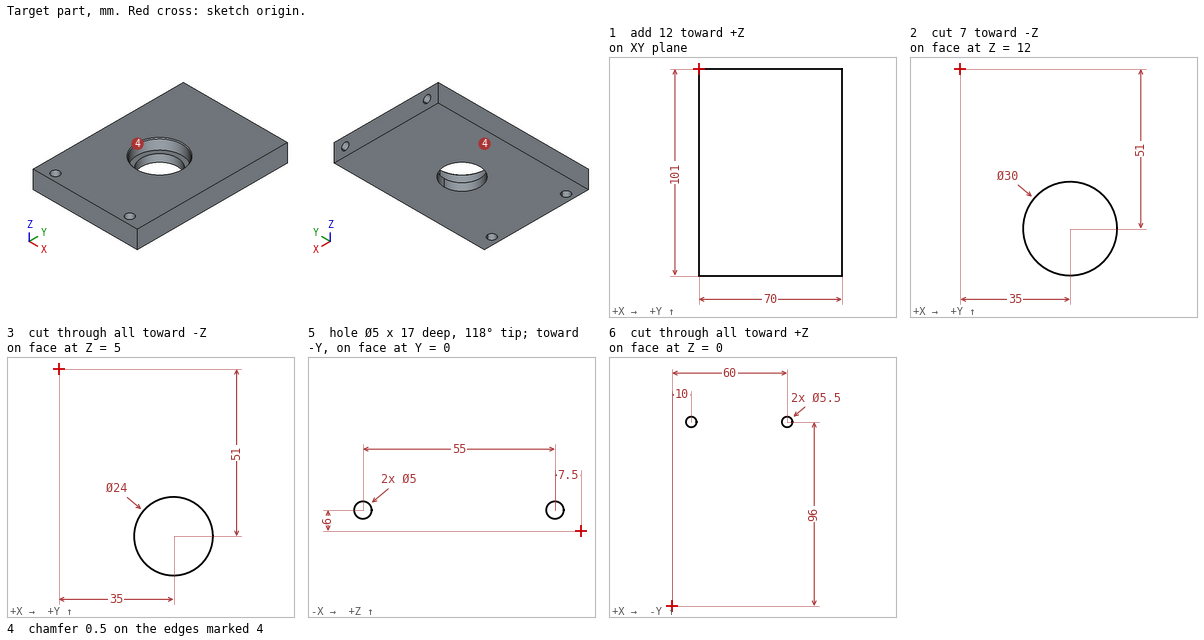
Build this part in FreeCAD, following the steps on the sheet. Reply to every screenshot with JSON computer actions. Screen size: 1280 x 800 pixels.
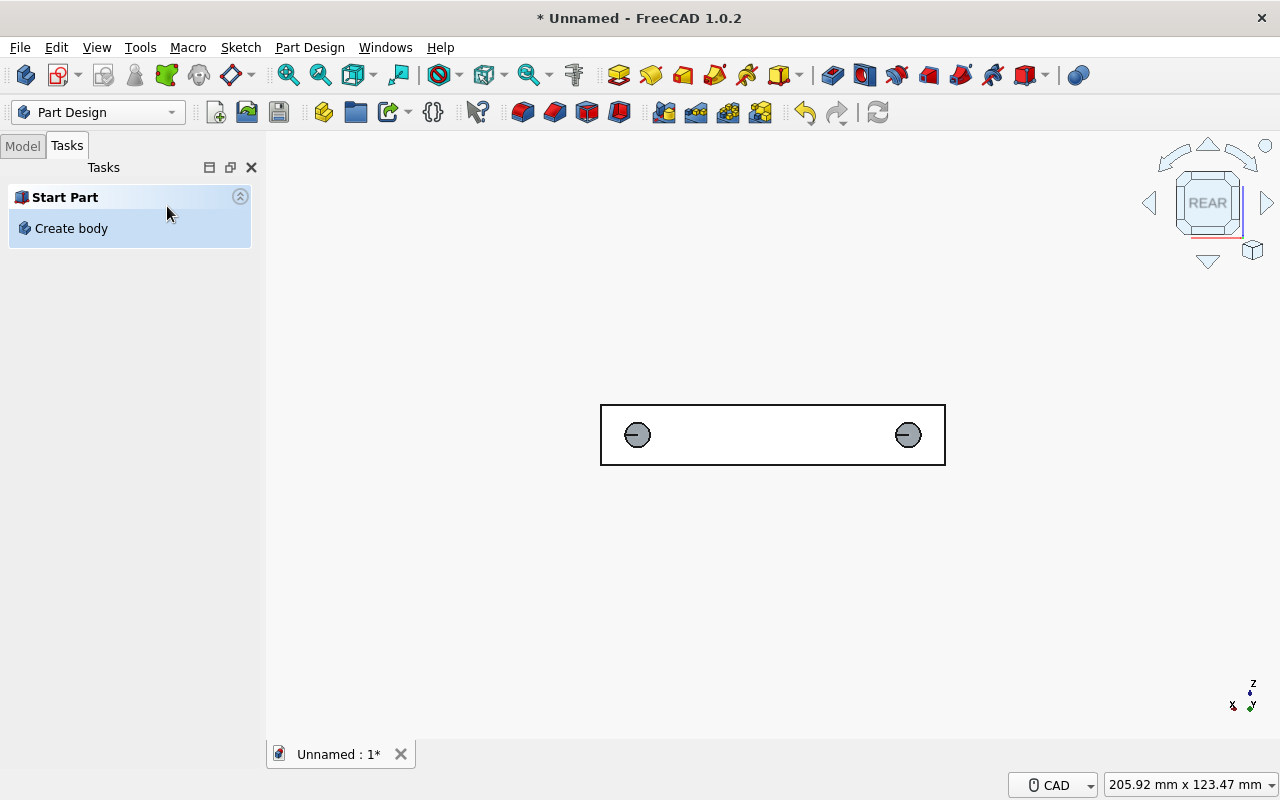
{"action": "left_click", "coordinate": [290, 76]}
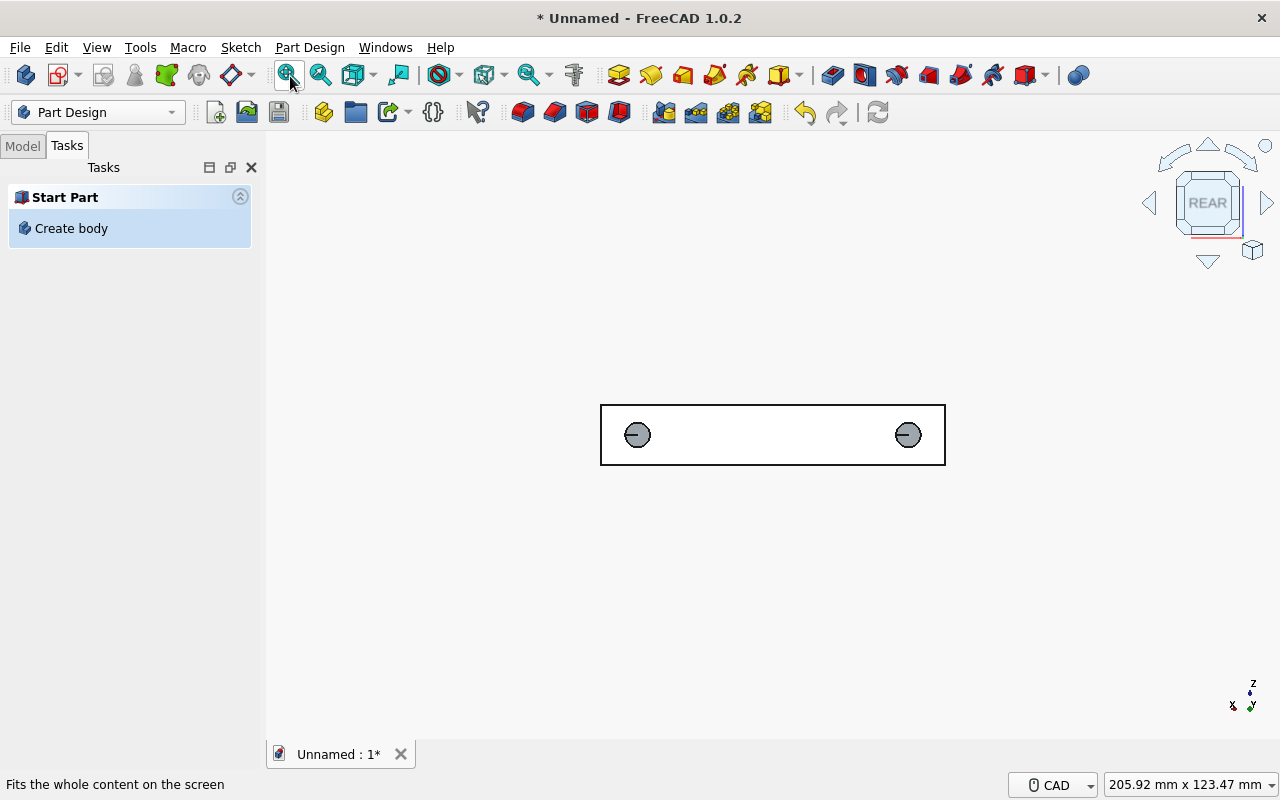
{"action": "key", "text": "5"}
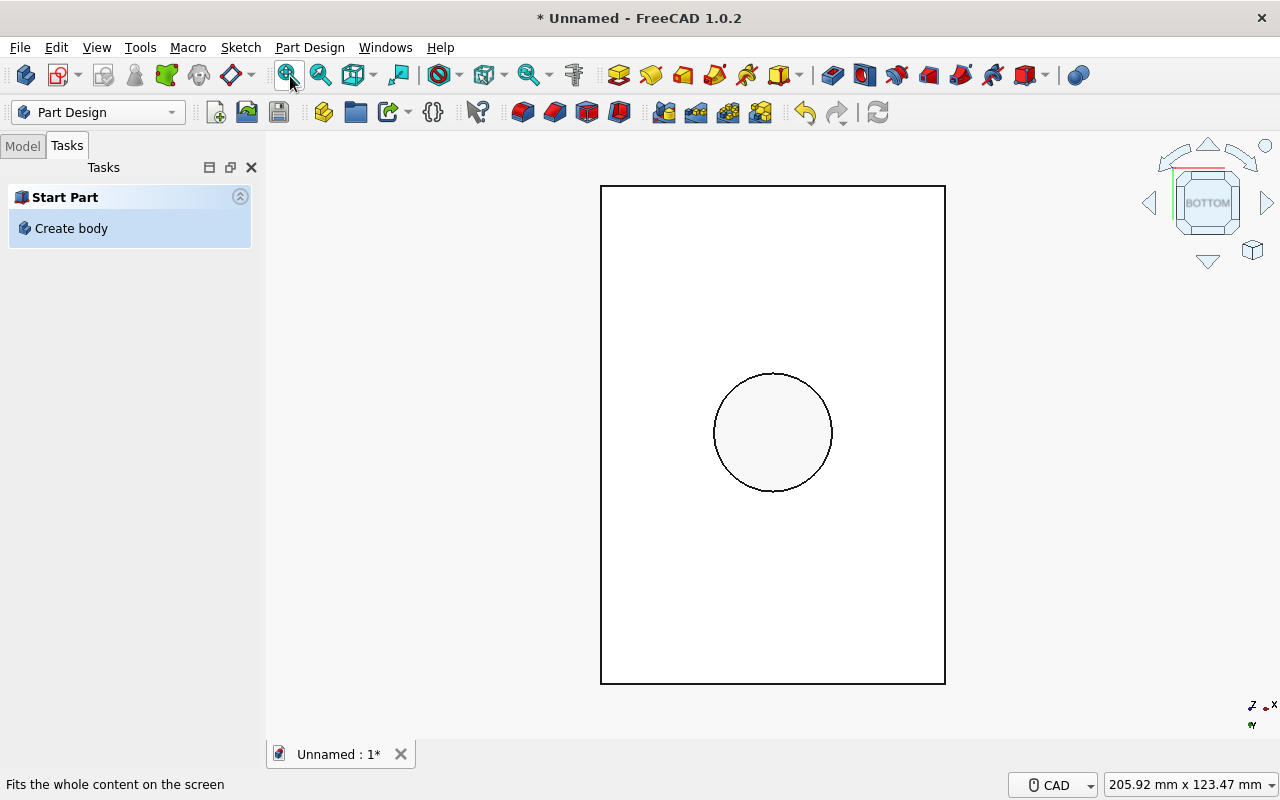
{"action": "left_click", "coordinate": [822, 576]}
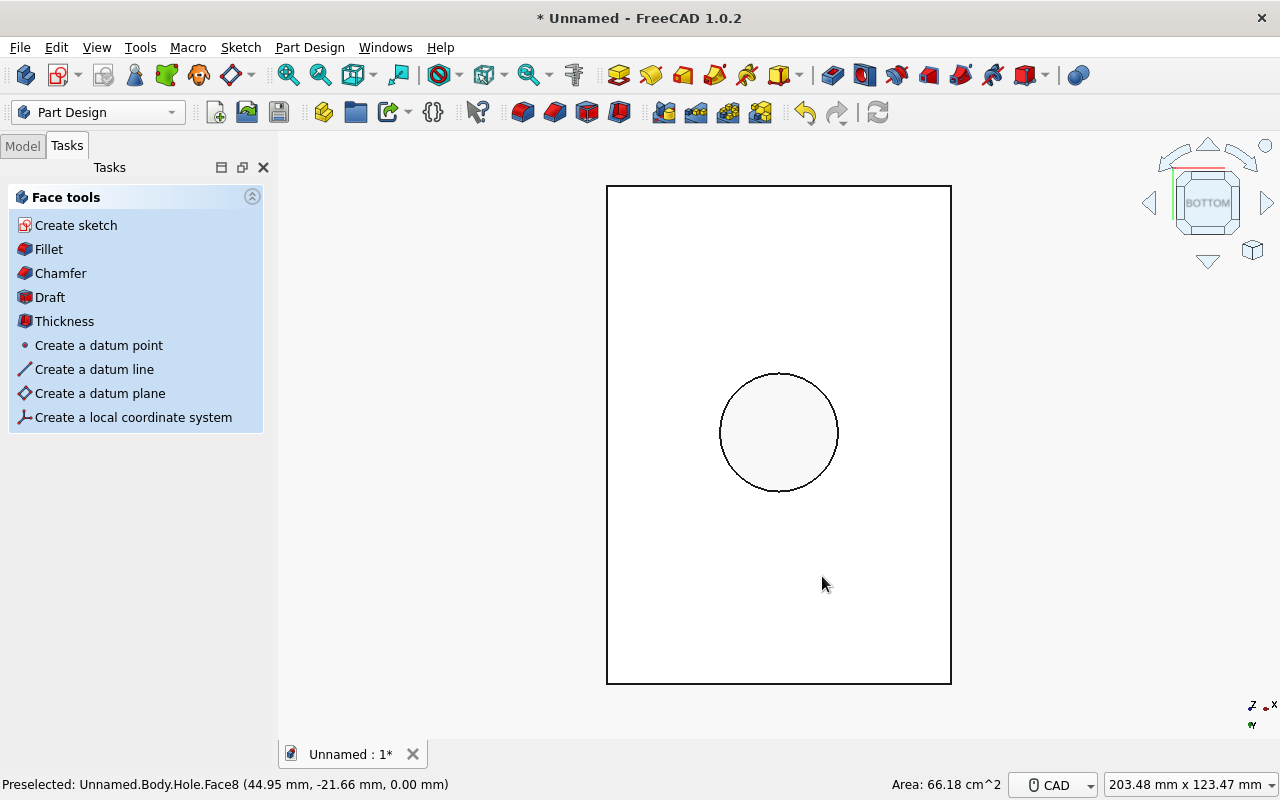
{"action": "left_click", "coordinate": [58, 76]}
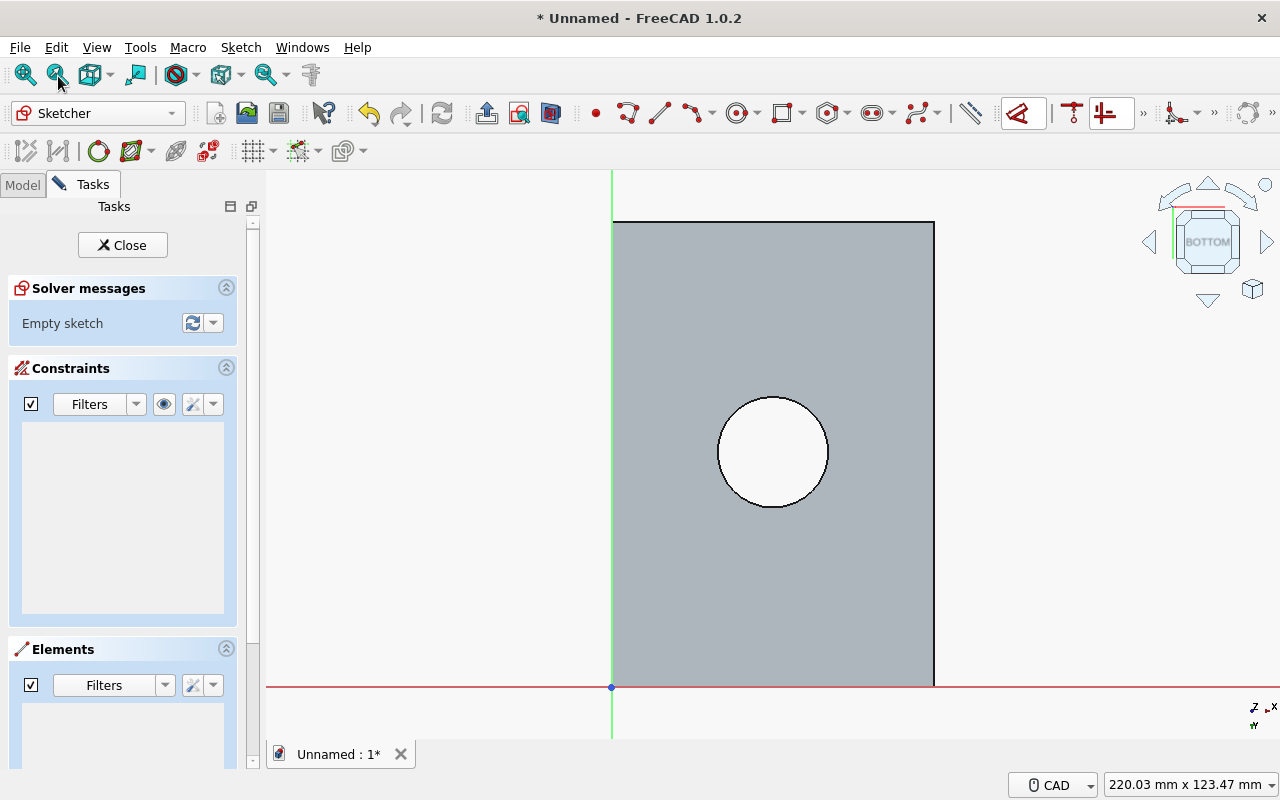
{"action": "scroll", "coordinate": [471, 431], "scroll_direction": "down", "scroll_amount": 1}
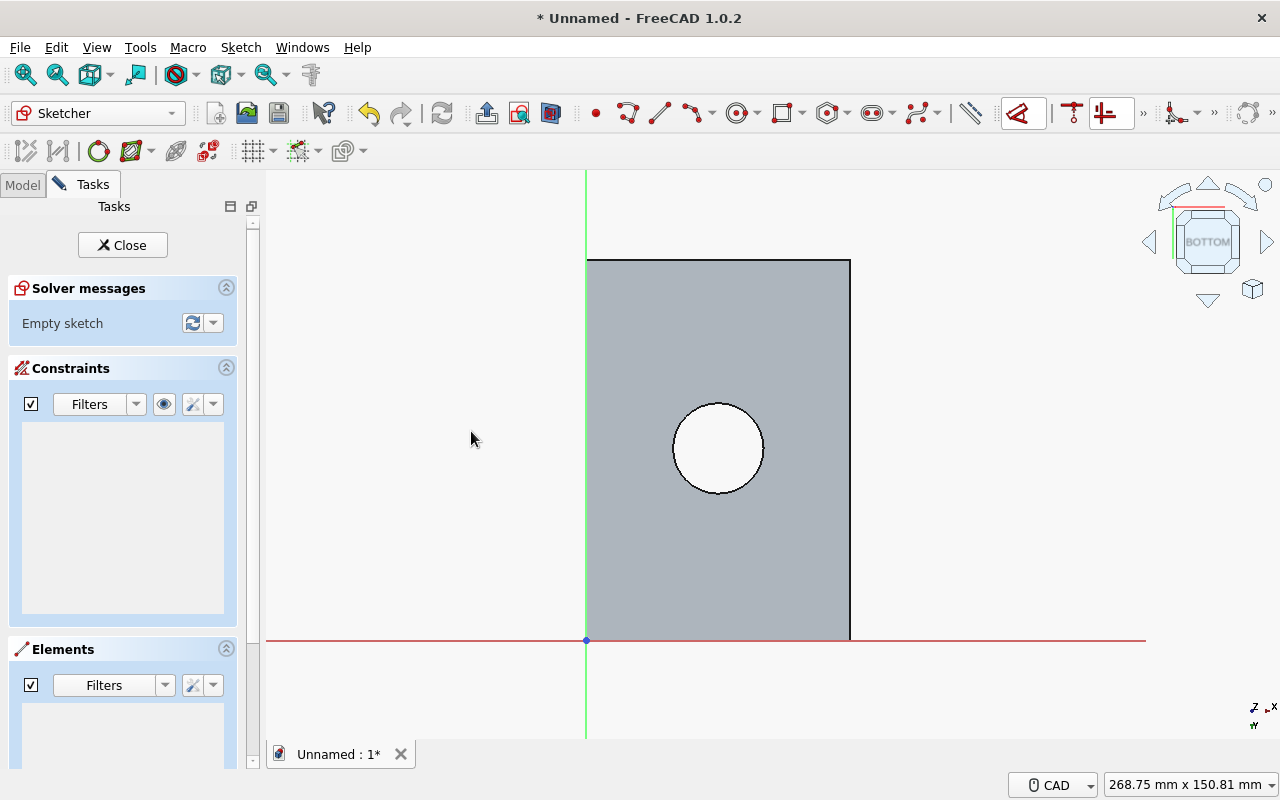
{"action": "key", "text": "g c"}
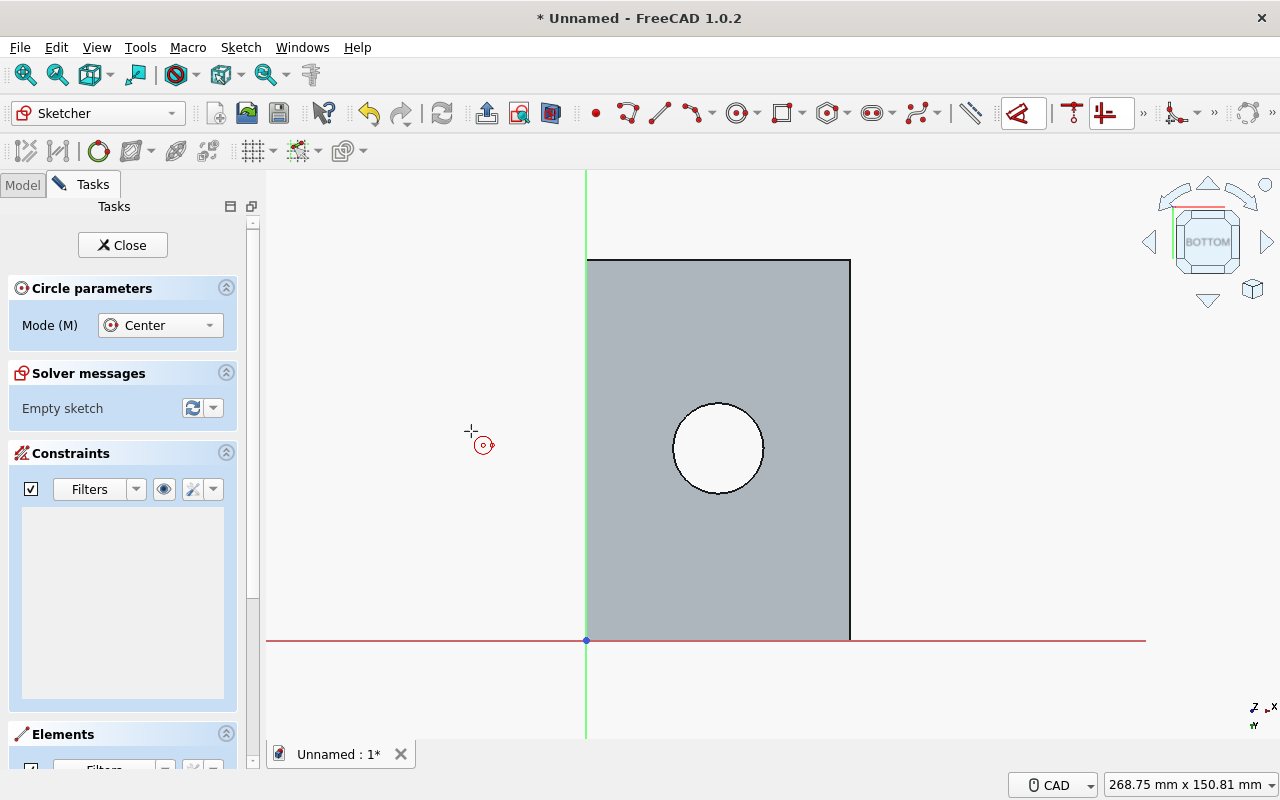
{"action": "scroll", "coordinate": [813, 279], "scroll_direction": "up", "scroll_amount": 4}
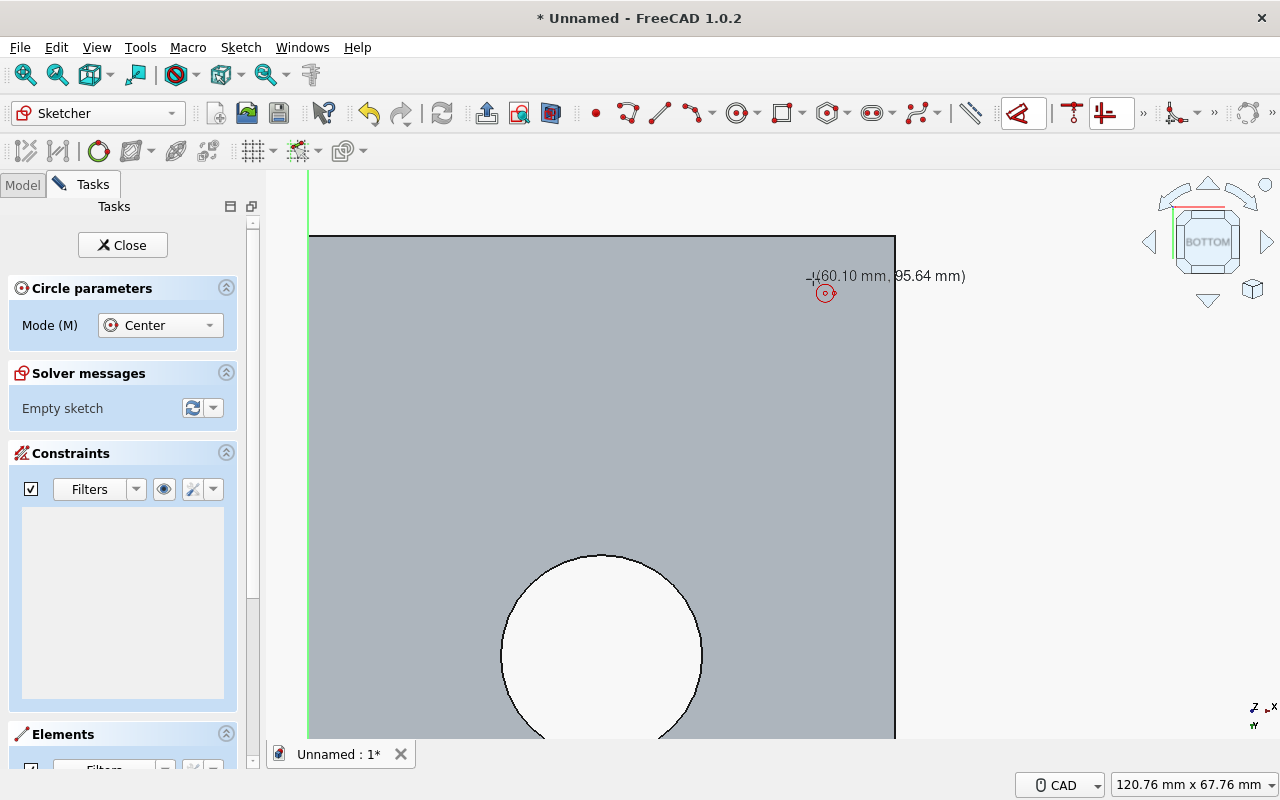
{"action": "left_click", "coordinate": [811, 278]}
{"action": "left_click", "coordinate": [828, 262]}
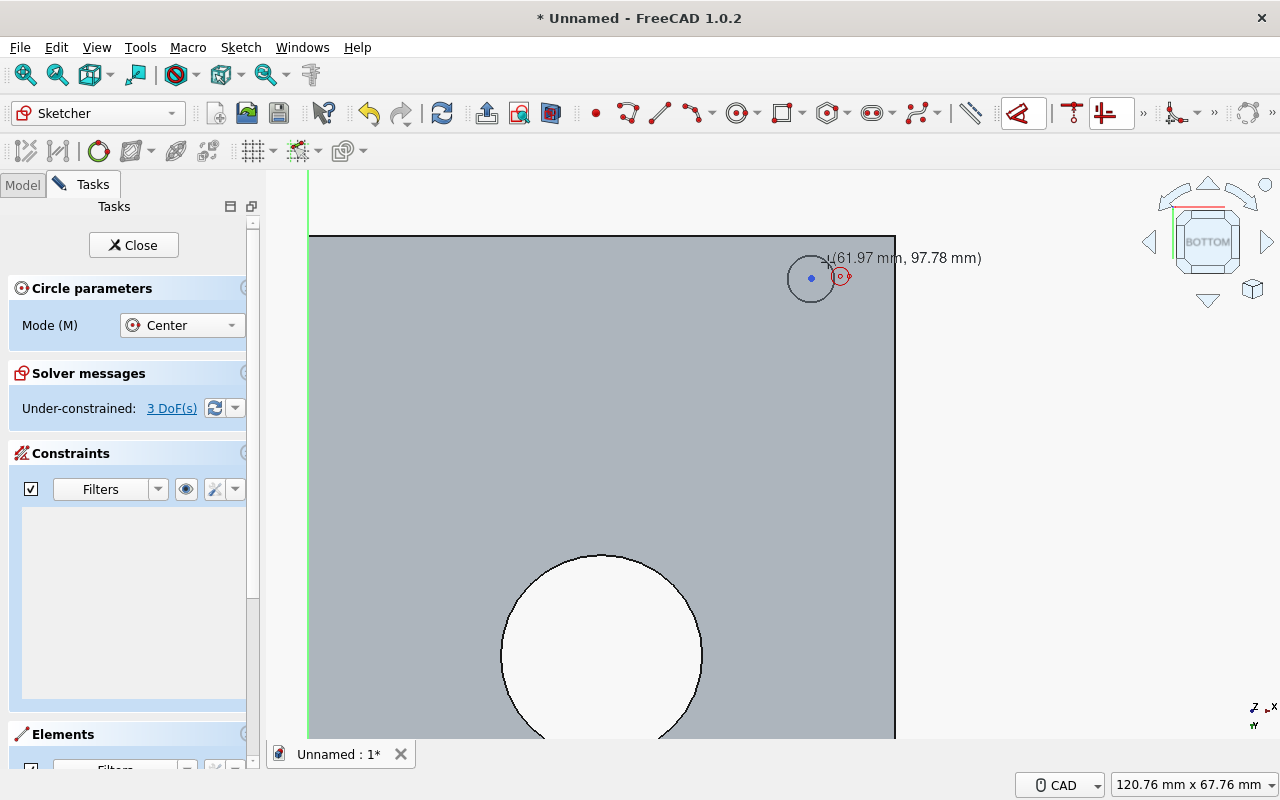
{"action": "left_click", "coordinate": [392, 278]}
{"action": "left_click", "coordinate": [408, 262]}
{"action": "key", "text": "Escape"}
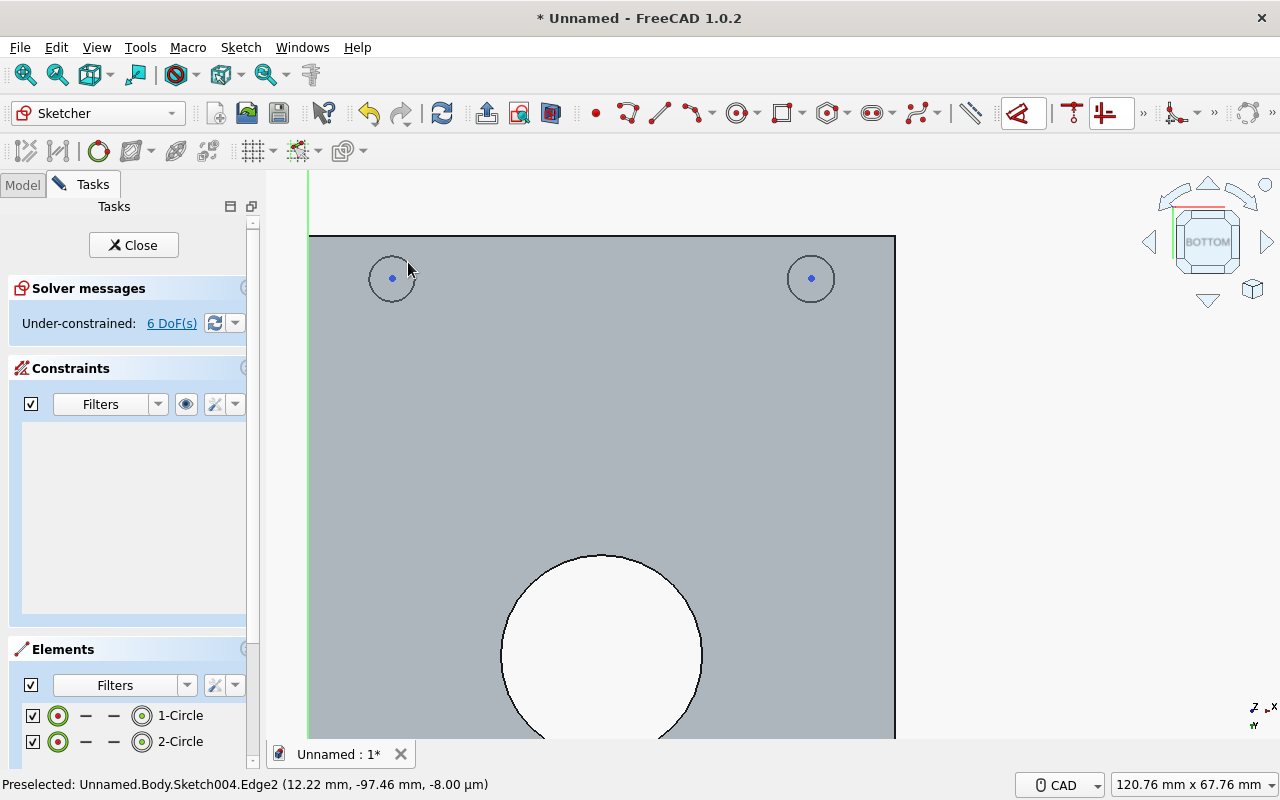
{"action": "left_click", "coordinate": [827, 262]}